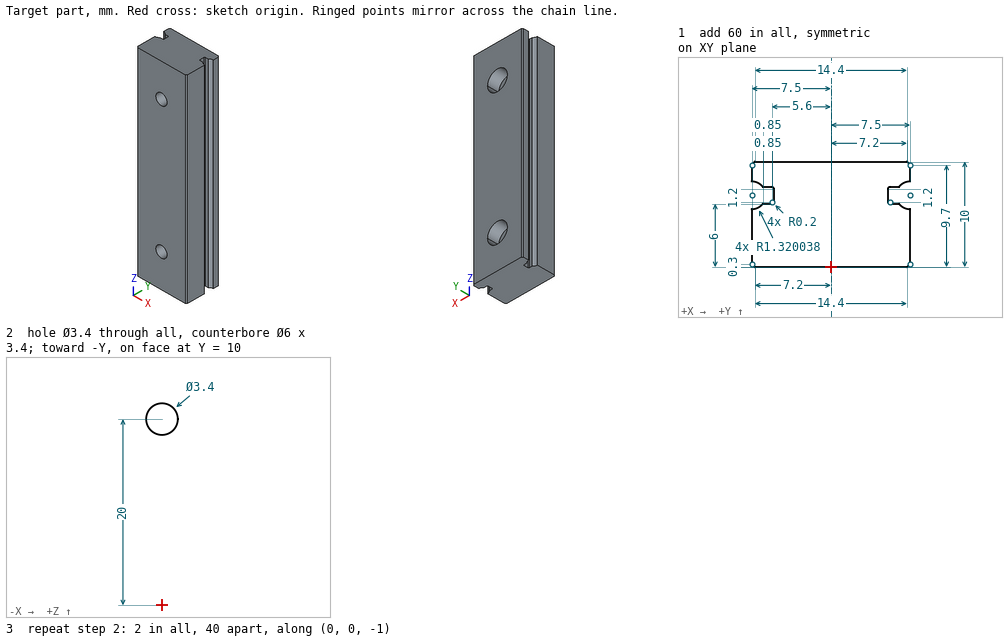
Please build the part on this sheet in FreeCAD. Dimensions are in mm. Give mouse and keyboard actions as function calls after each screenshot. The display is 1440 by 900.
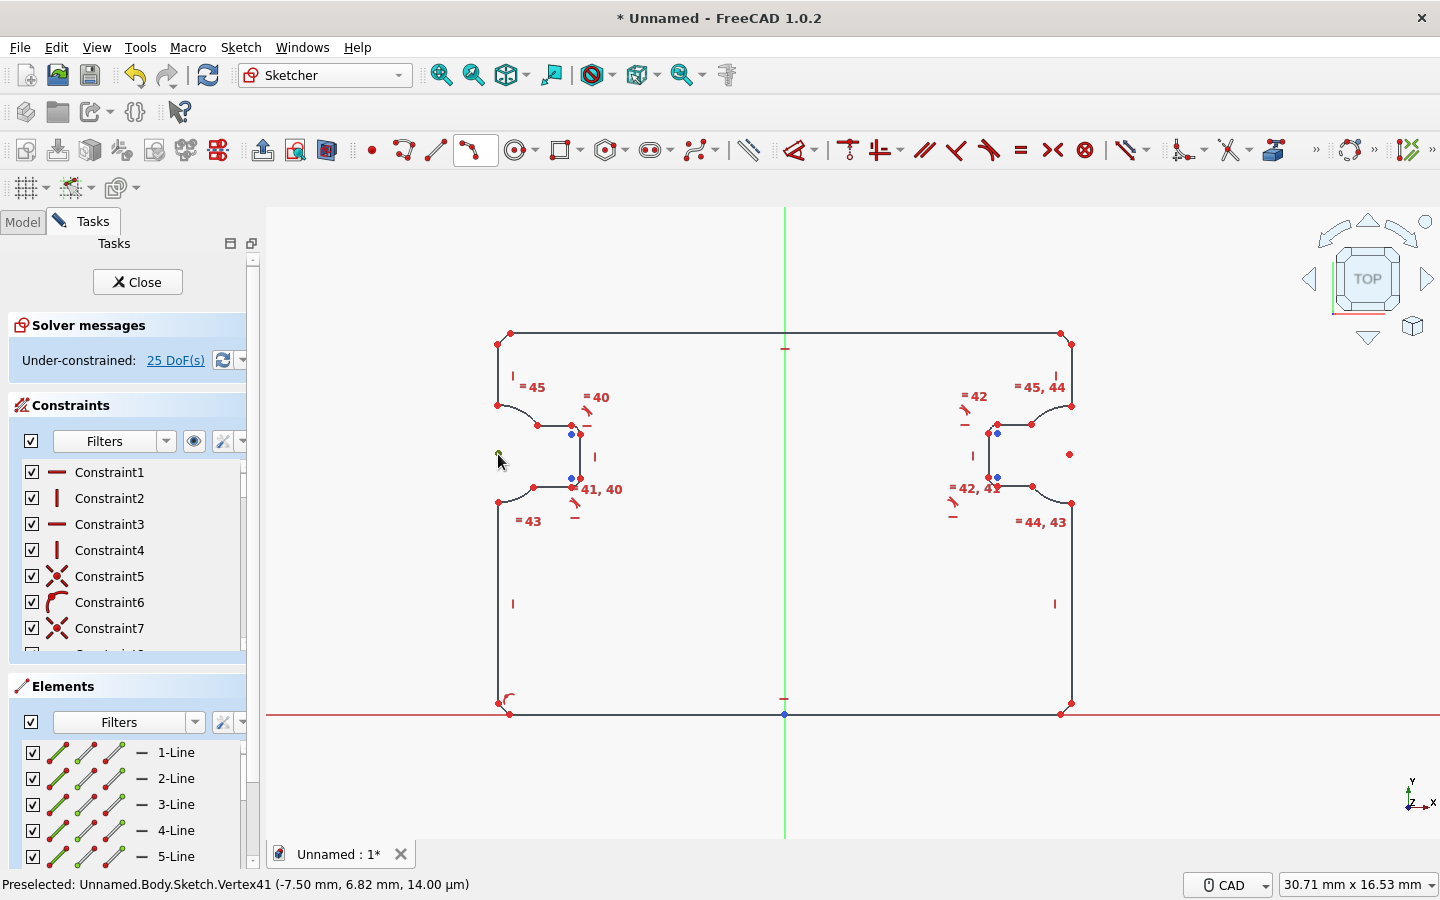
click(1070, 455)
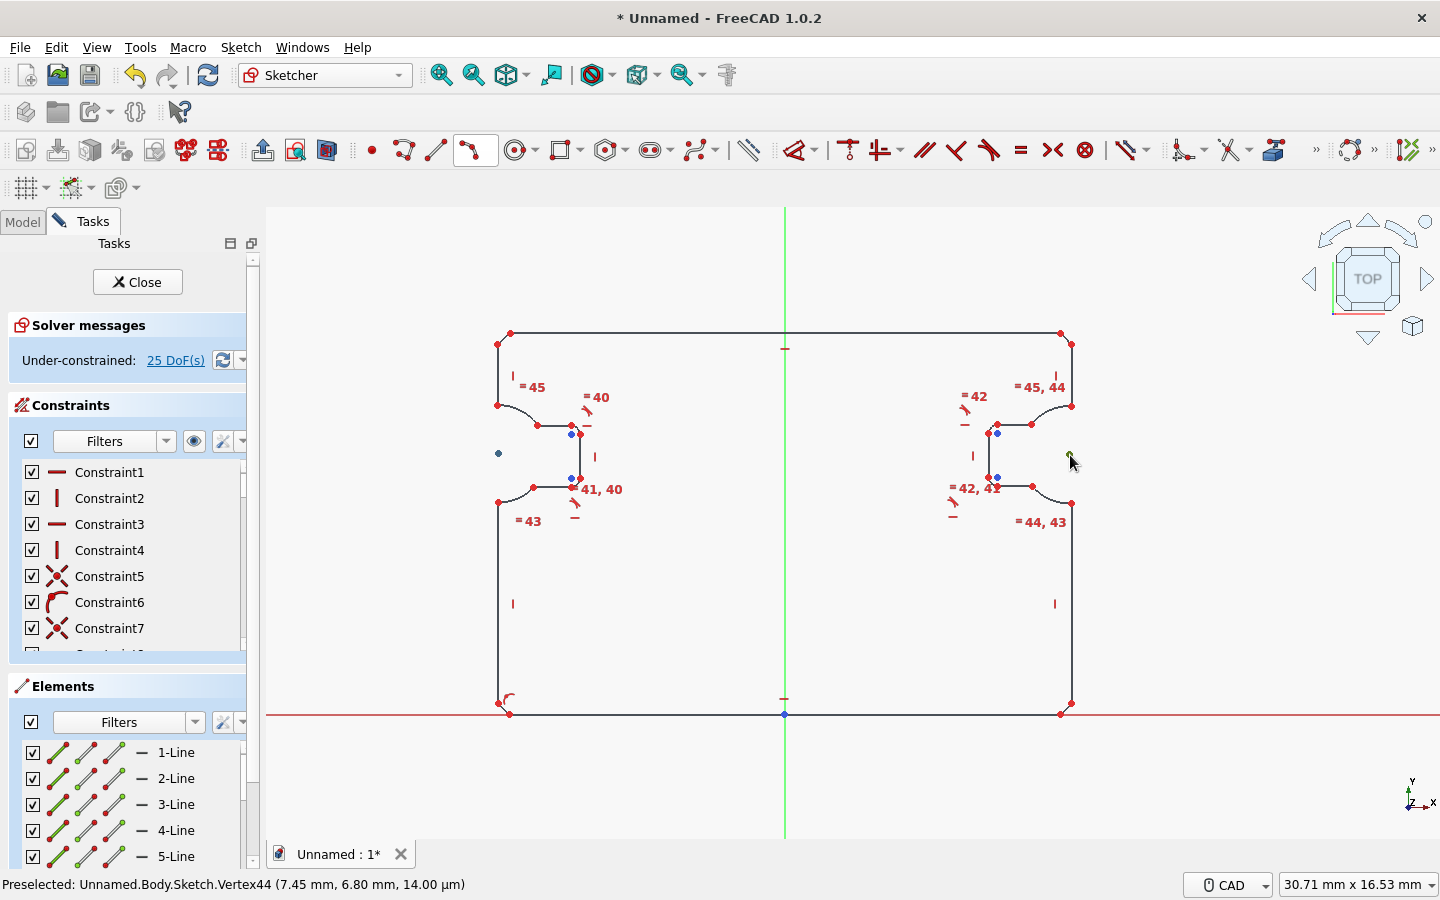
click(785, 770)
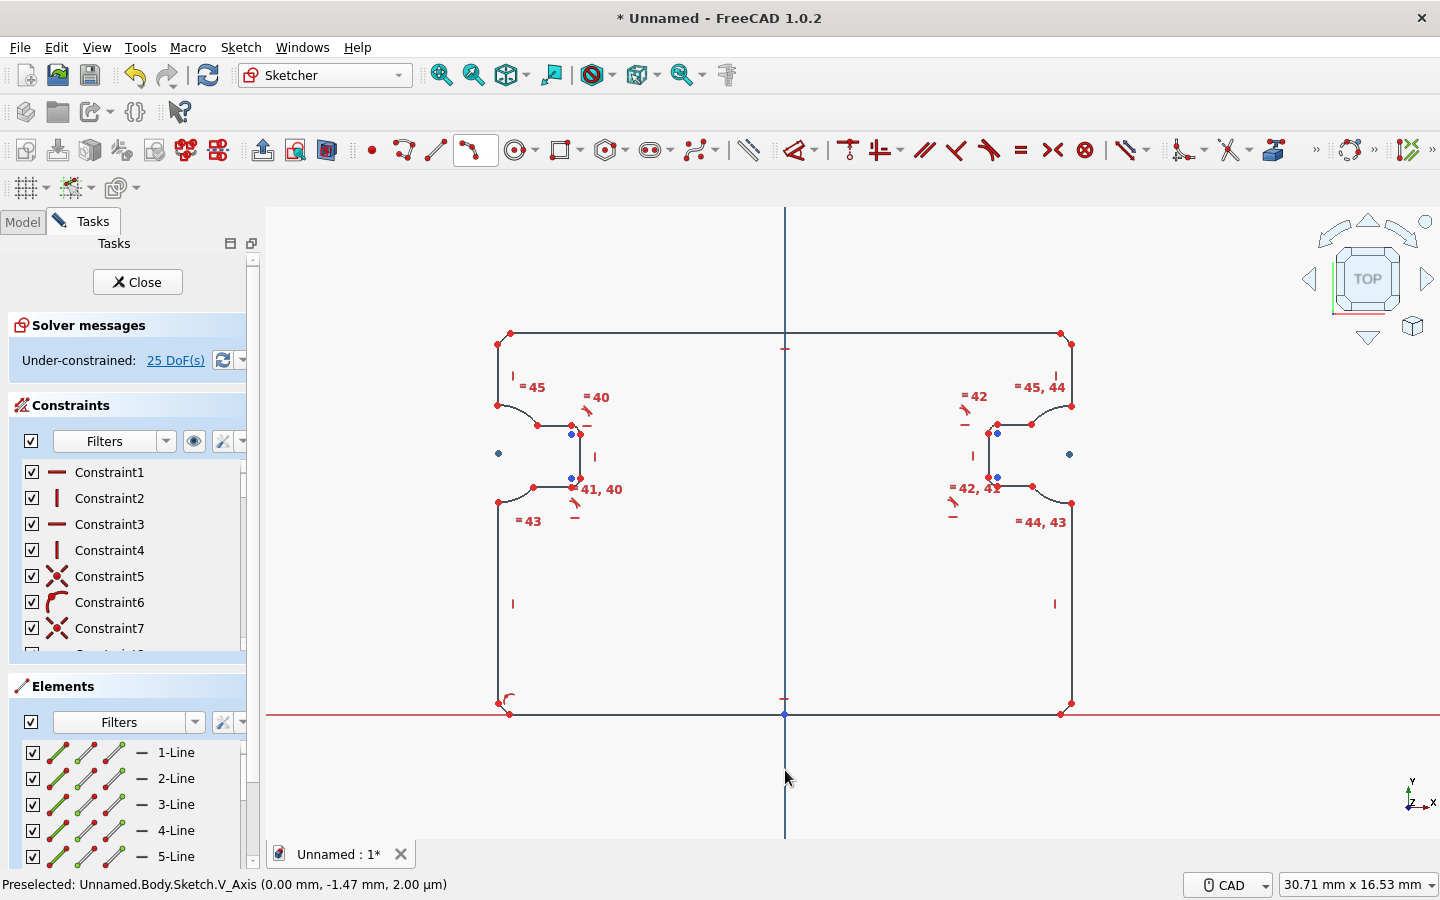
click(1054, 150)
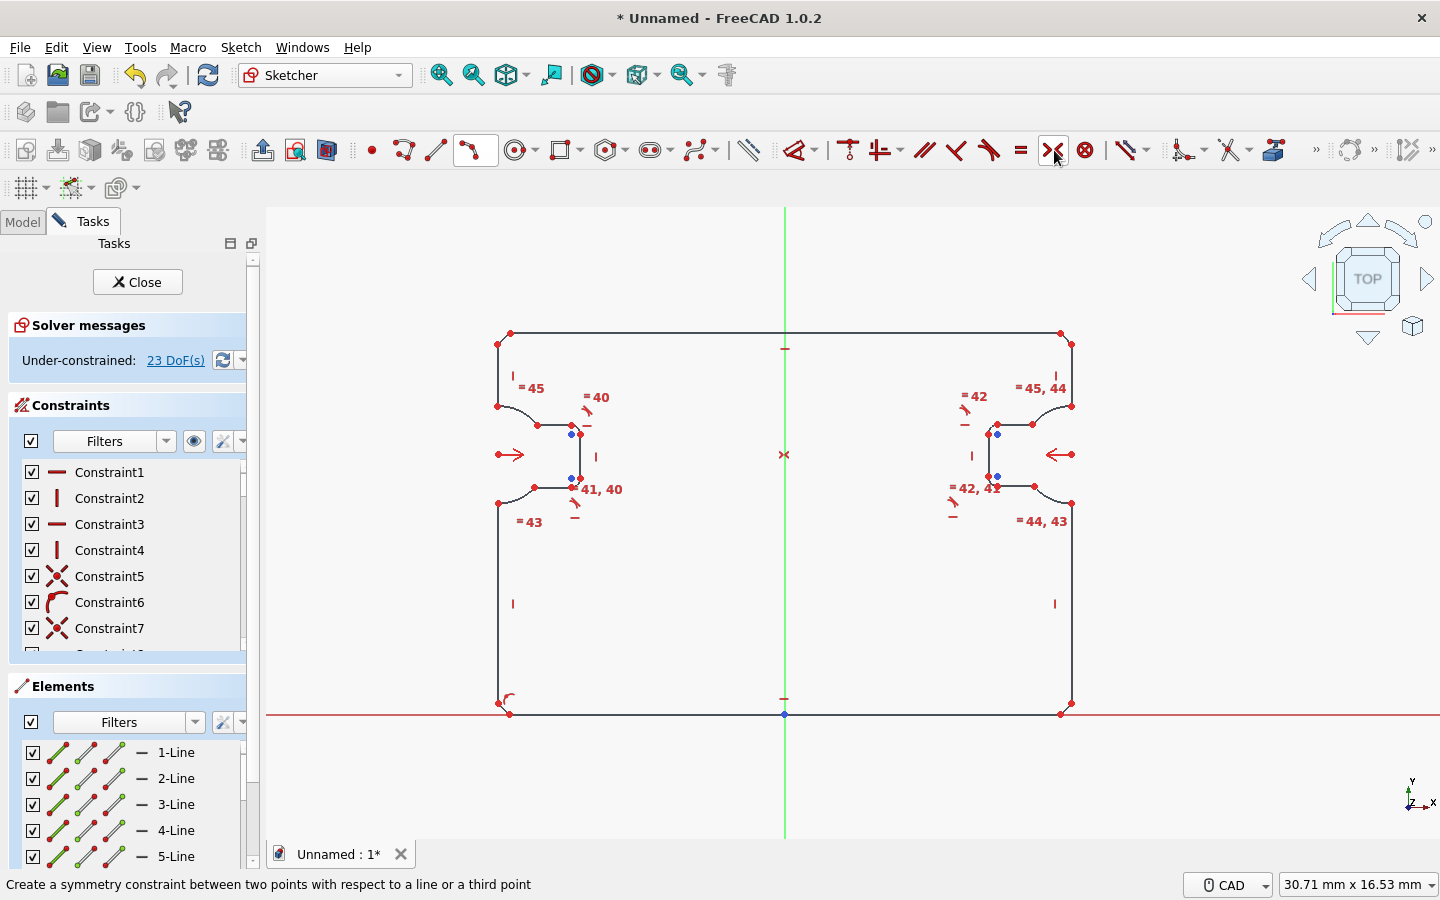
scroll(571, 478, up, 2)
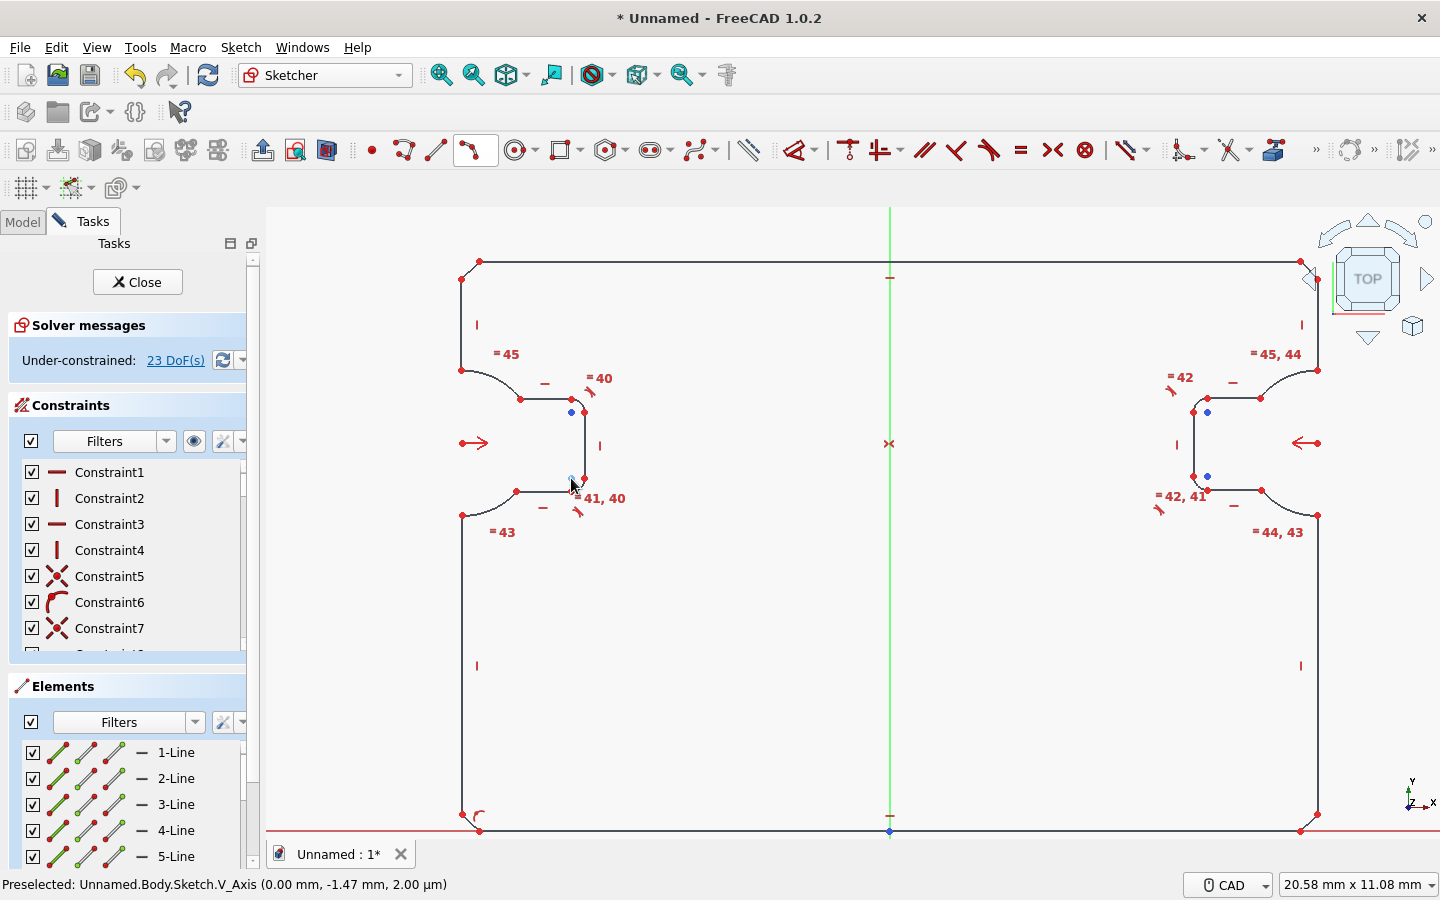
click(571, 478)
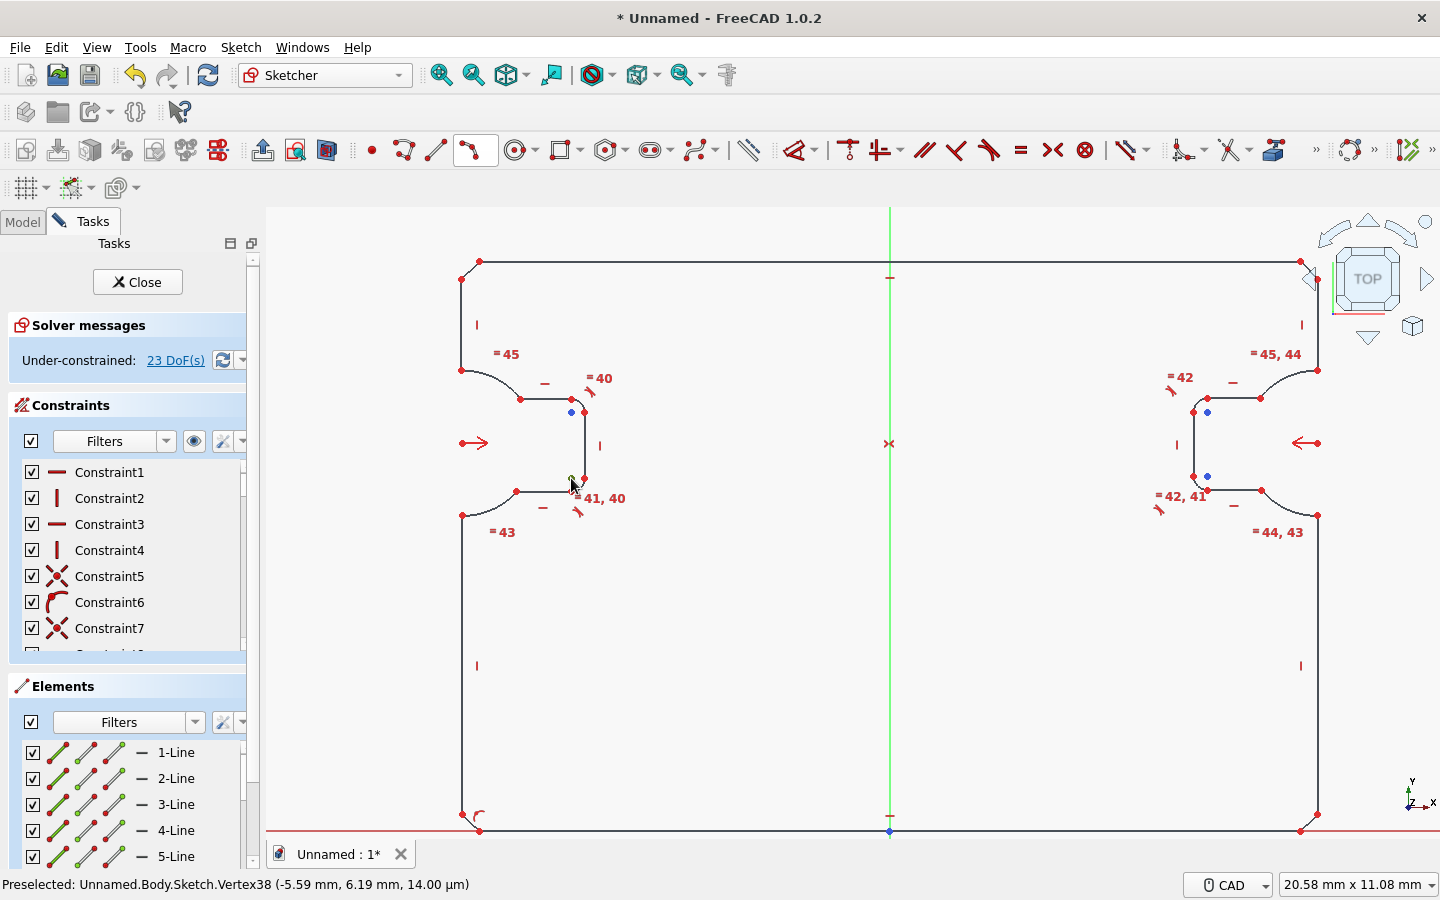
click(1208, 476)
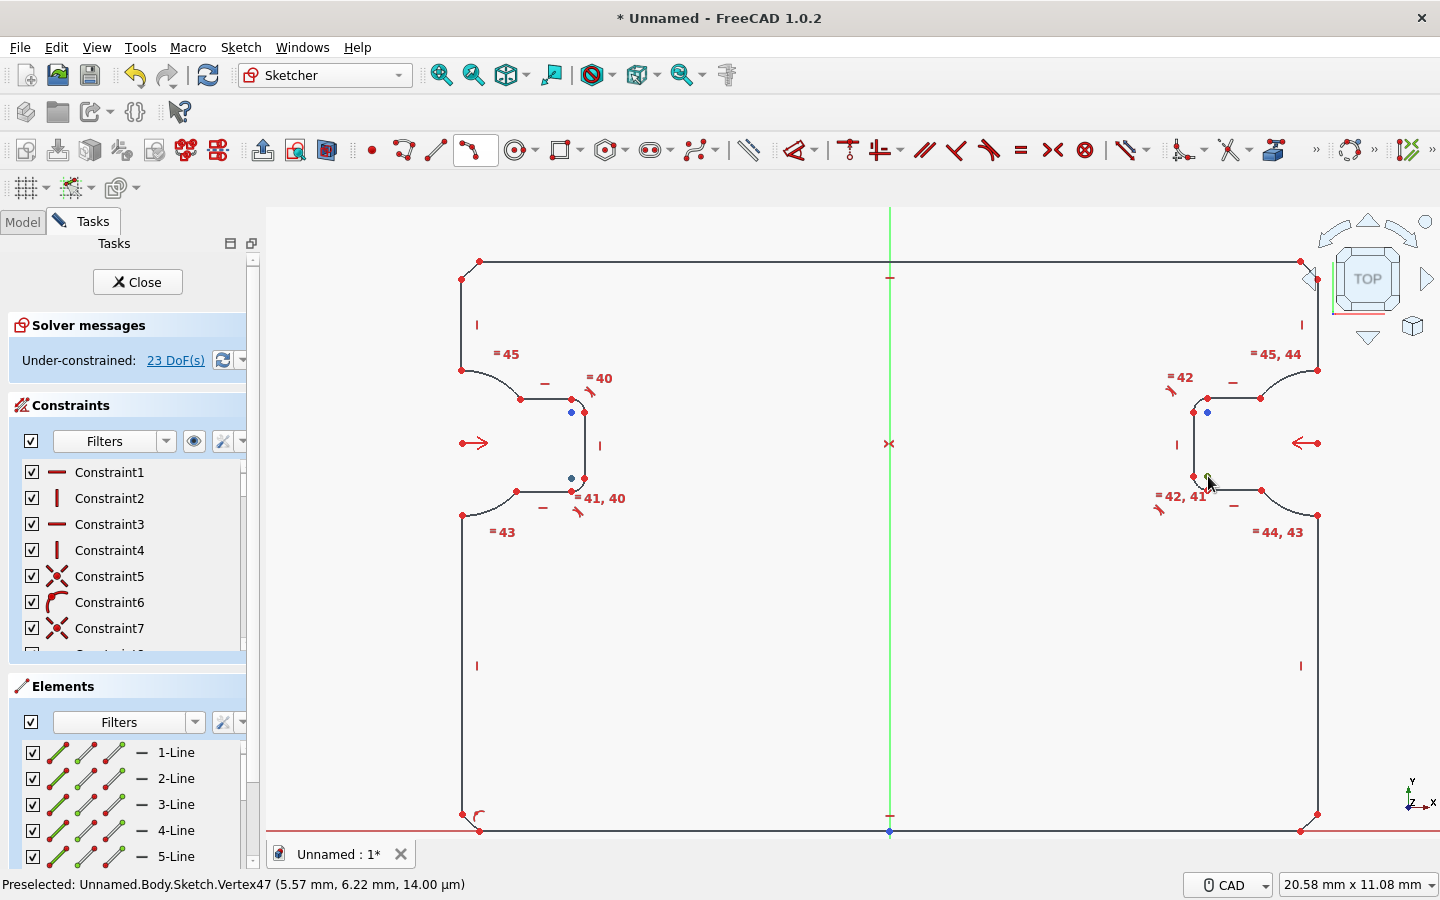
click(890, 770)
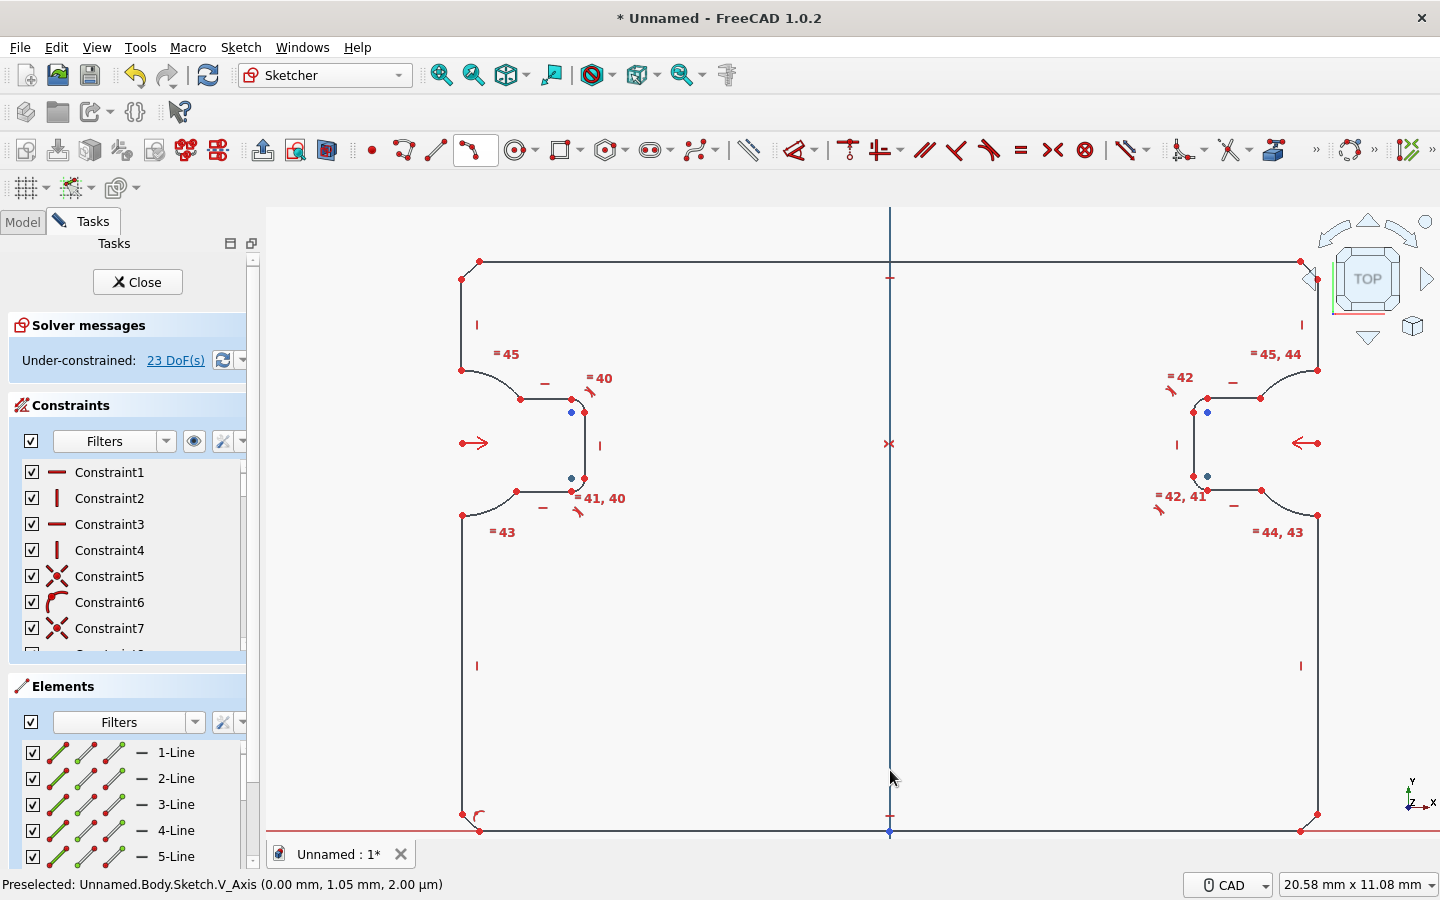
click(1054, 150)